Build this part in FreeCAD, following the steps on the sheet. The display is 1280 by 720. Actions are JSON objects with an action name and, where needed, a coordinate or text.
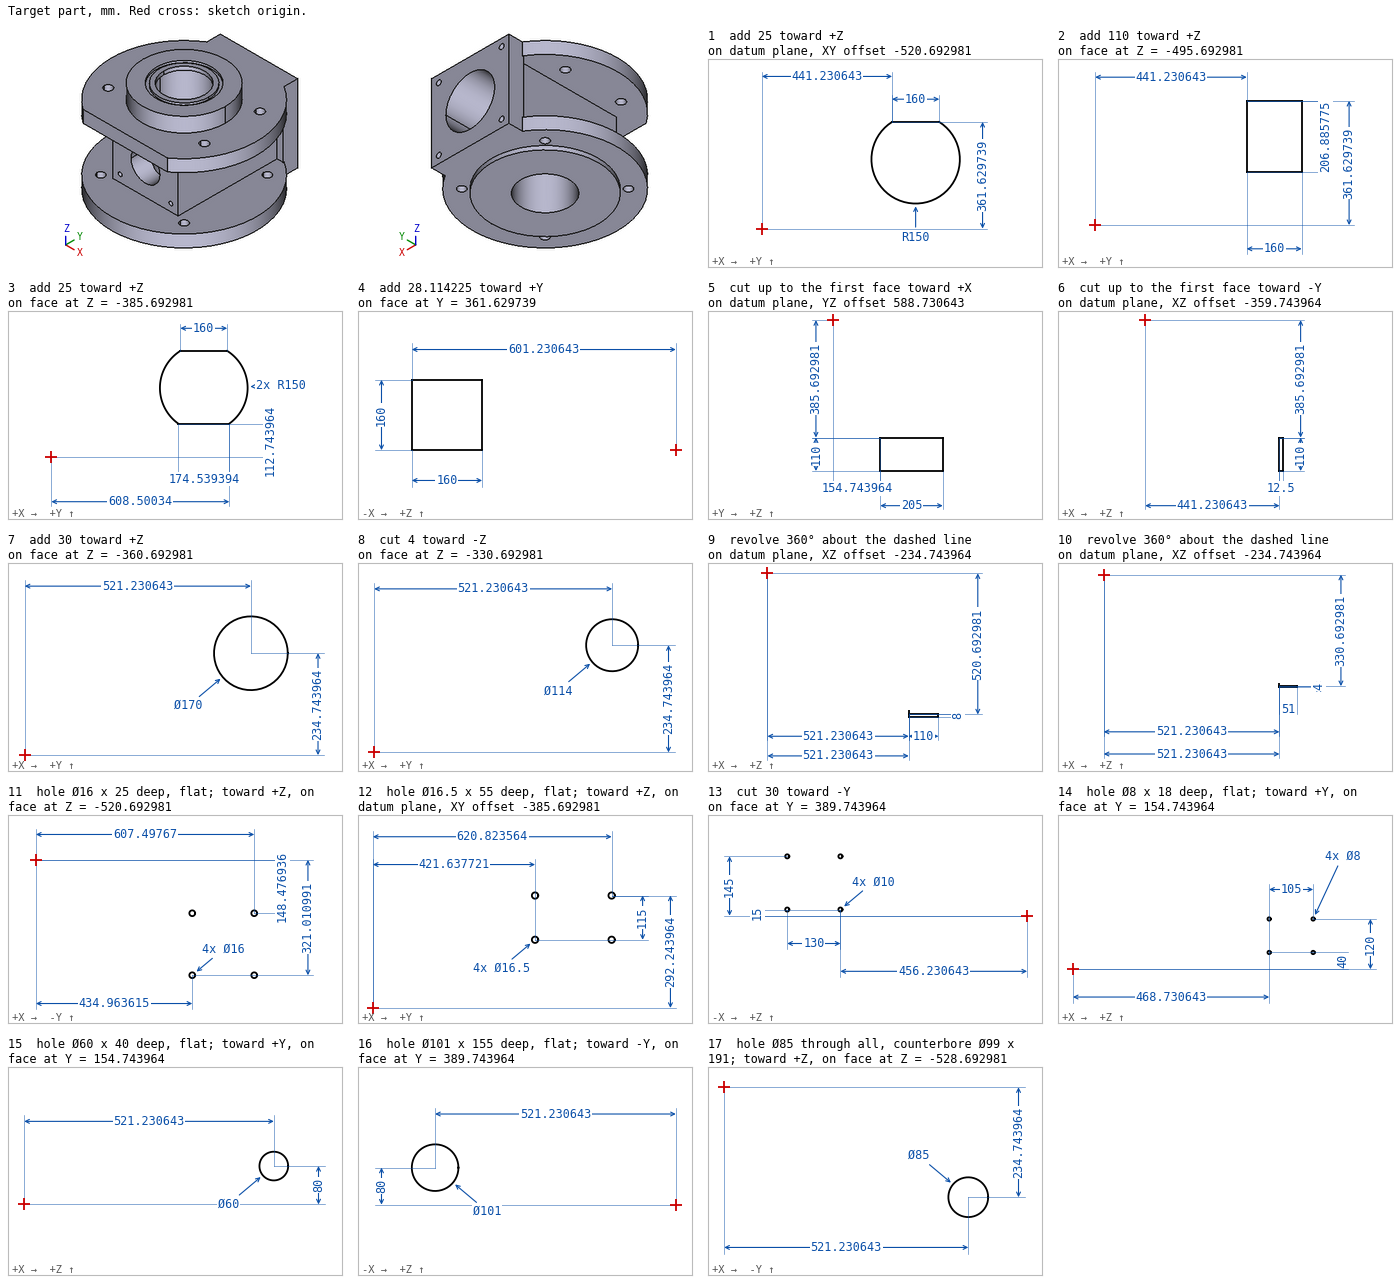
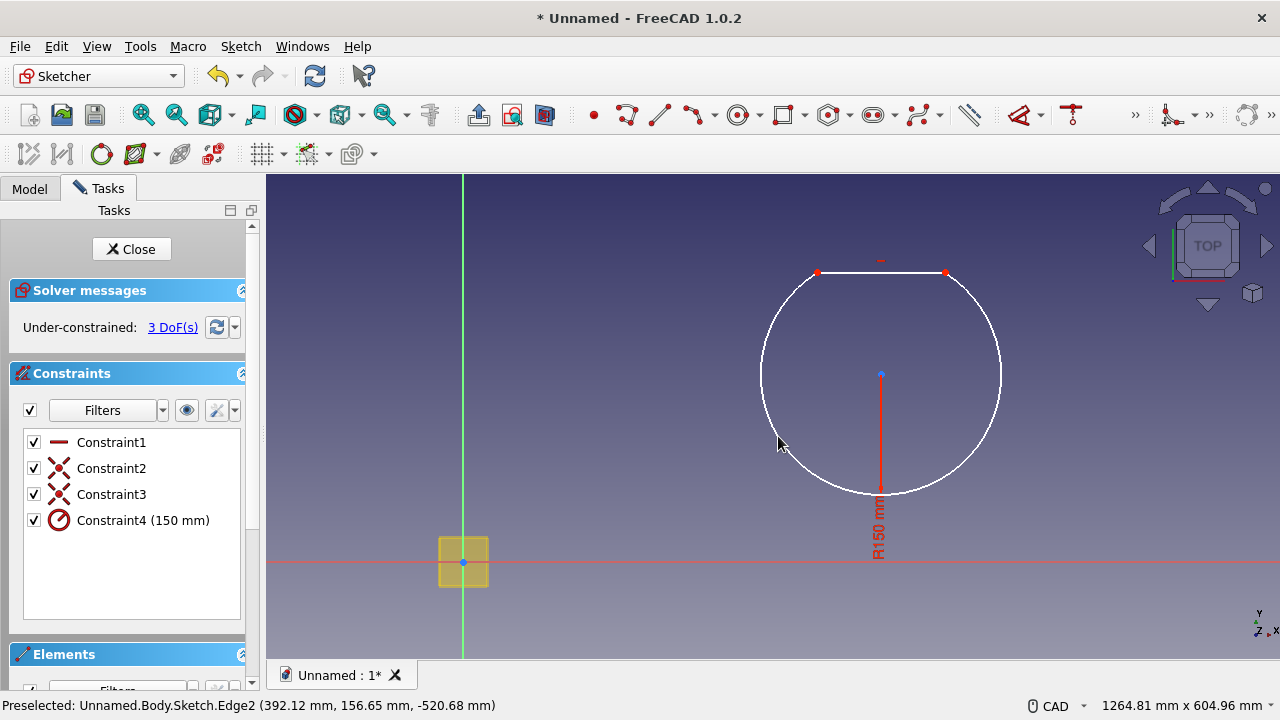
{"action": "left_click", "coordinate": [855, 273]}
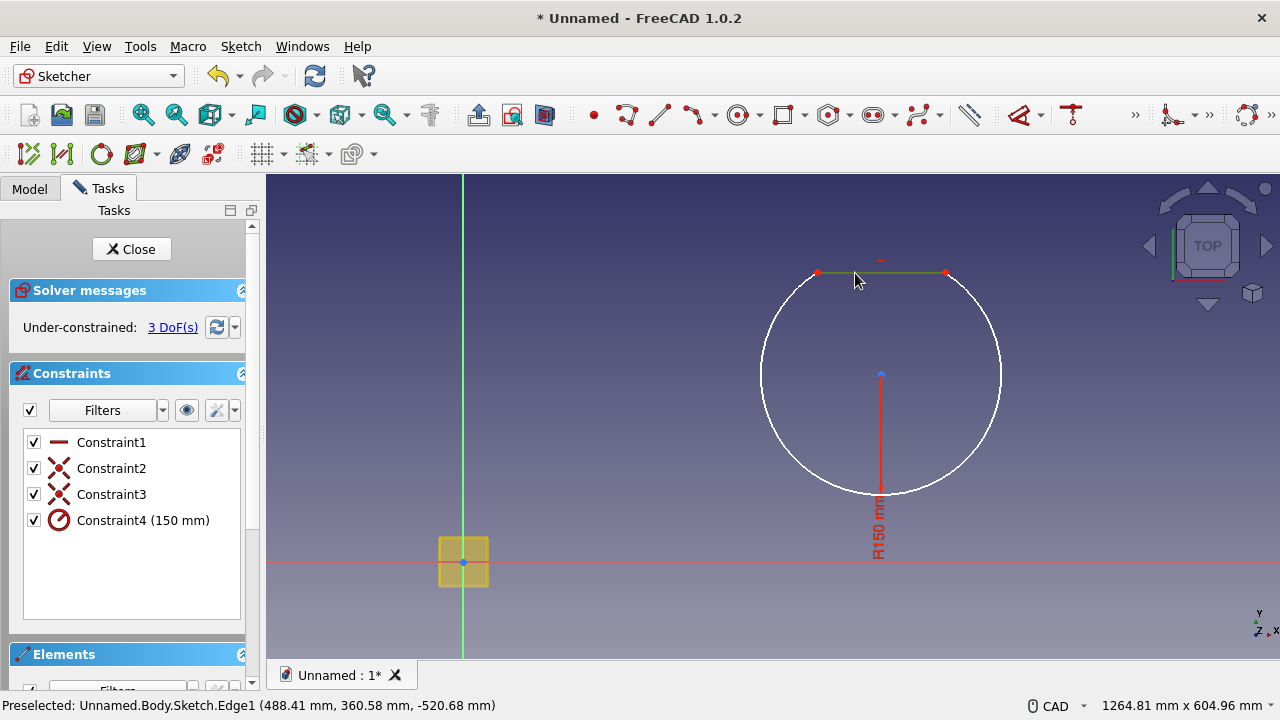
{"action": "left_click", "coordinate": [1040, 116]}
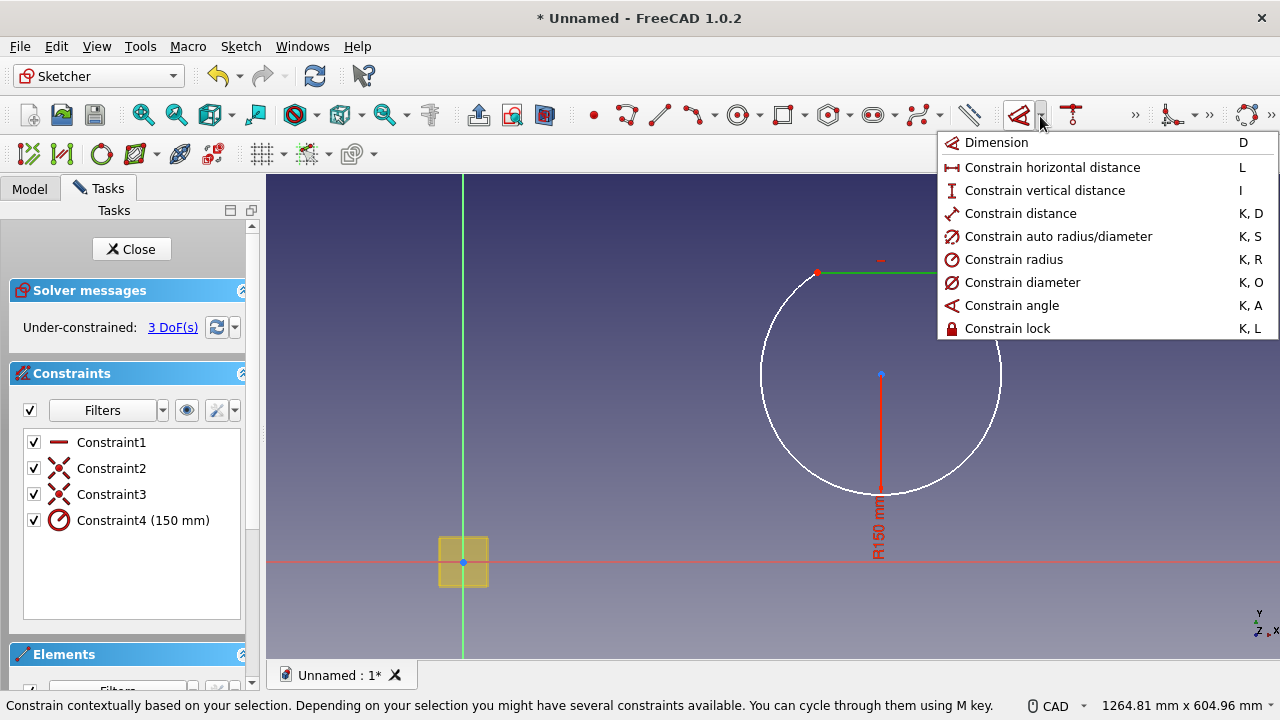
{"action": "left_click", "coordinate": [1108, 168]}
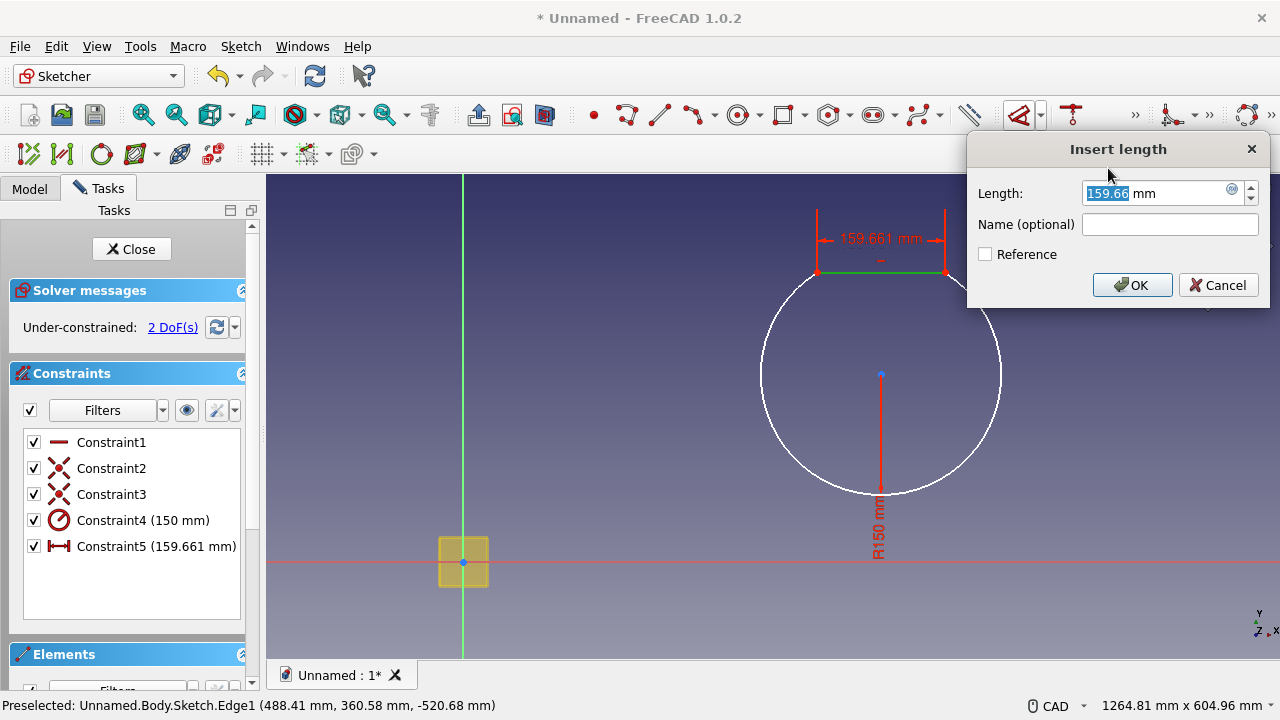
{"action": "type", "text": "160"}
{"action": "key", "text": "Return"}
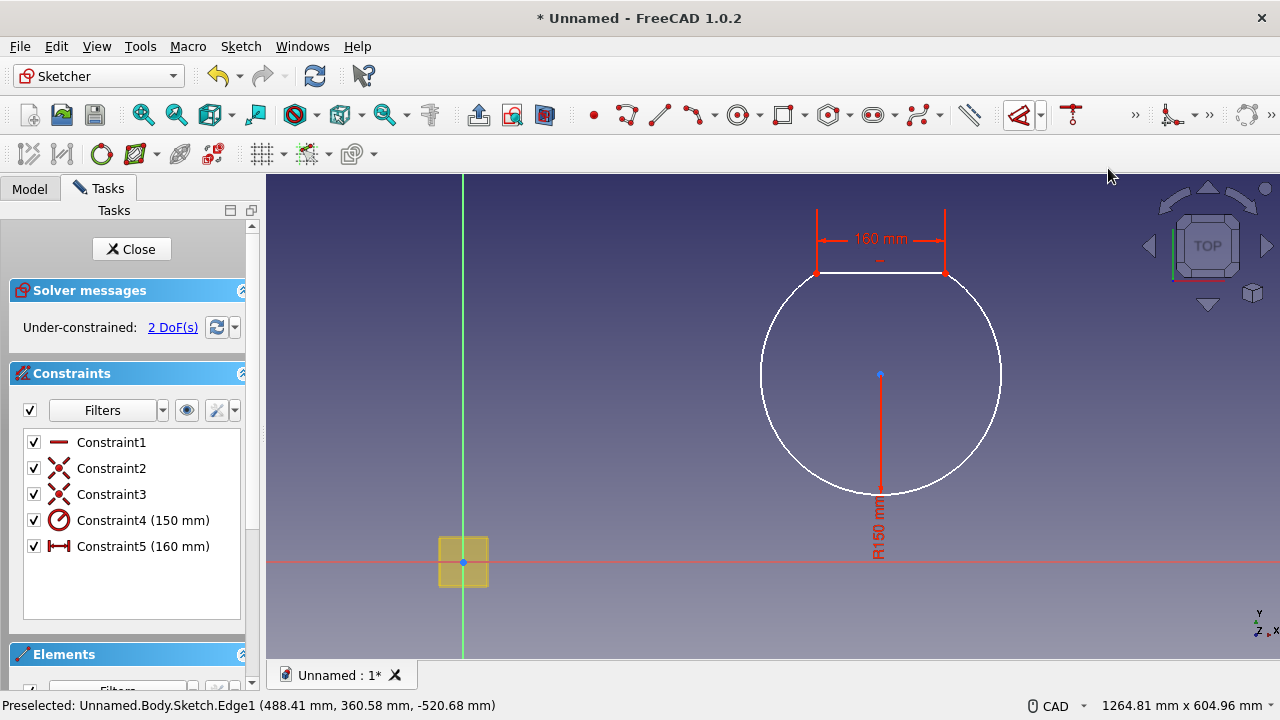
{"action": "left_click", "coordinate": [817, 273]}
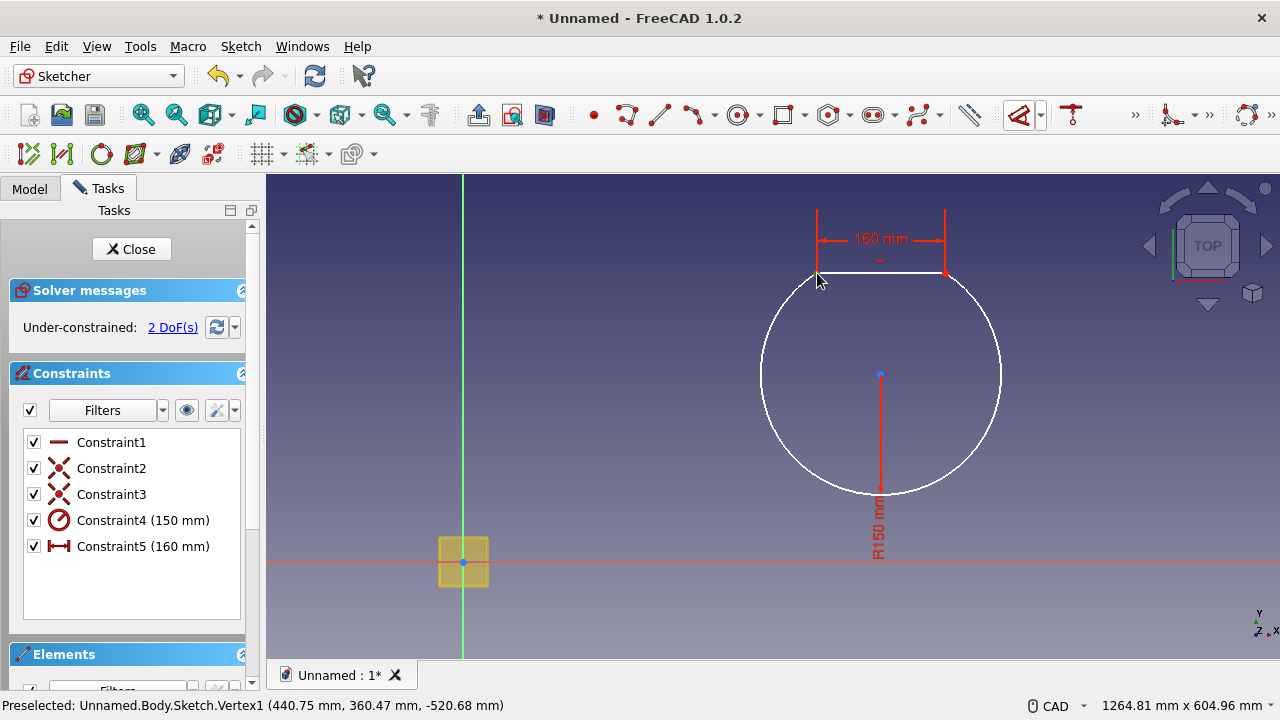
{"action": "left_click", "coordinate": [1040, 116]}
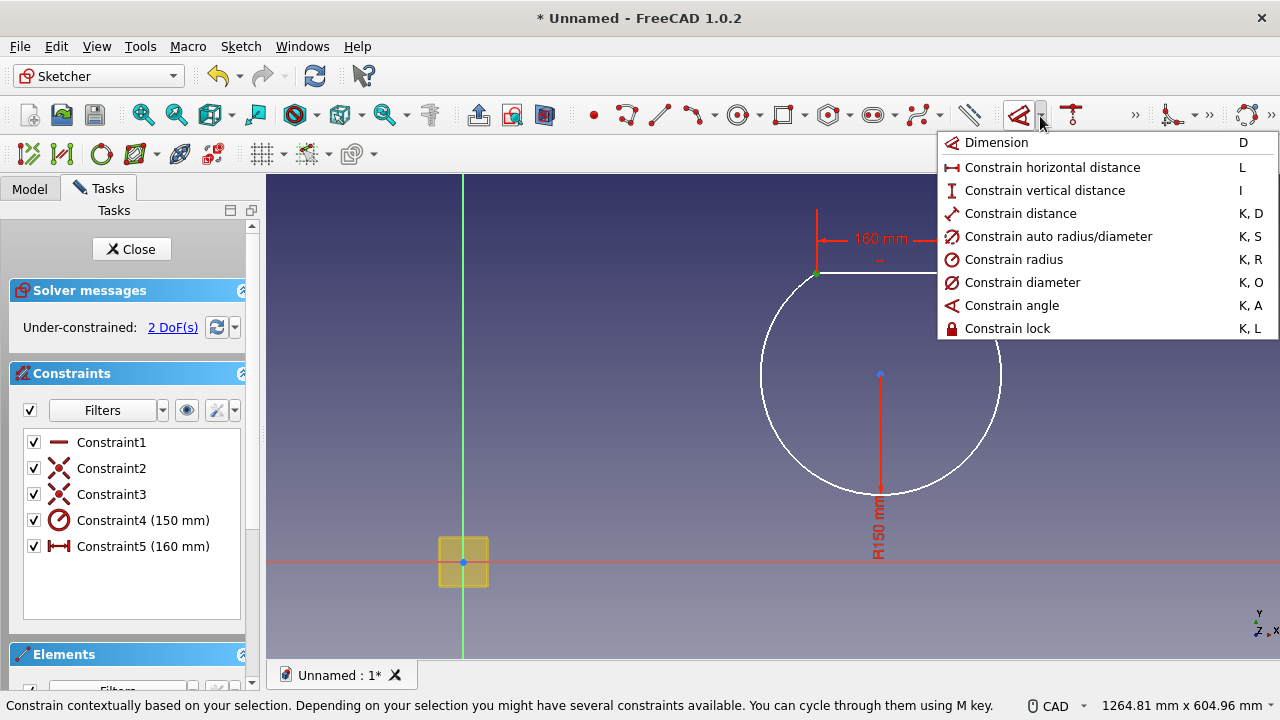
{"action": "left_click", "coordinate": [1108, 168]}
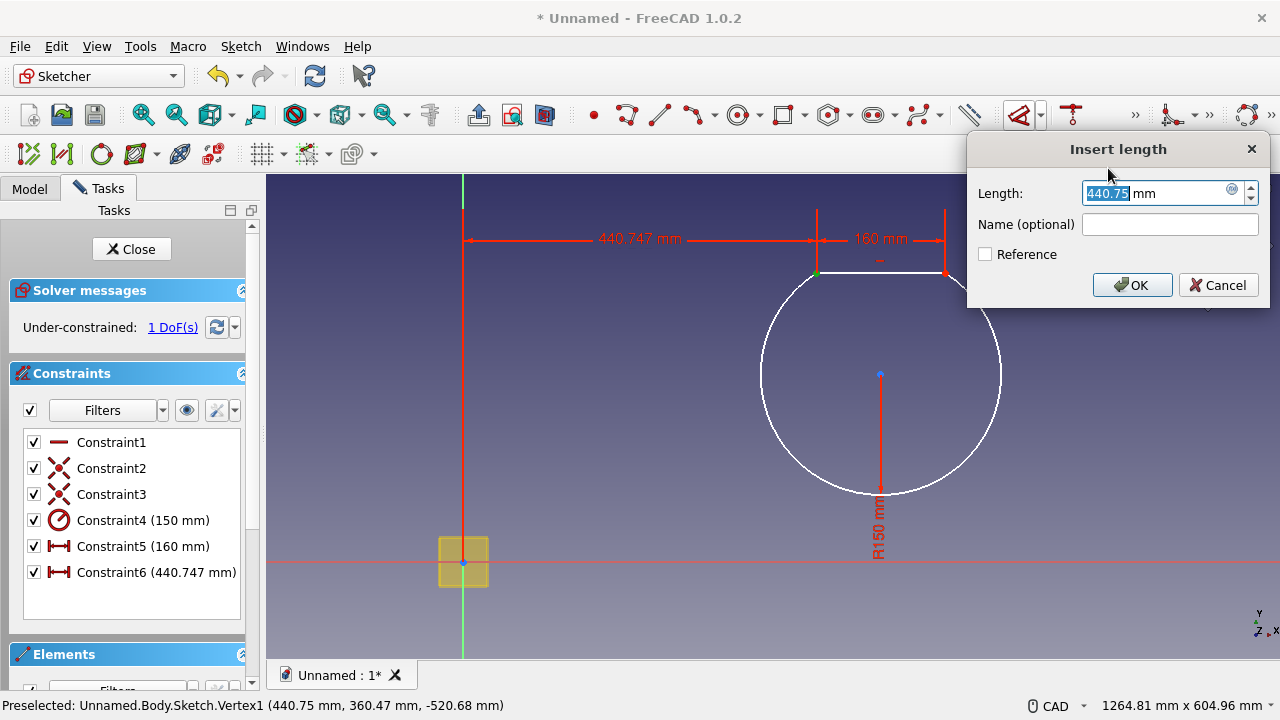
{"action": "type", "text": "441.230643"}
{"action": "key", "text": "Return"}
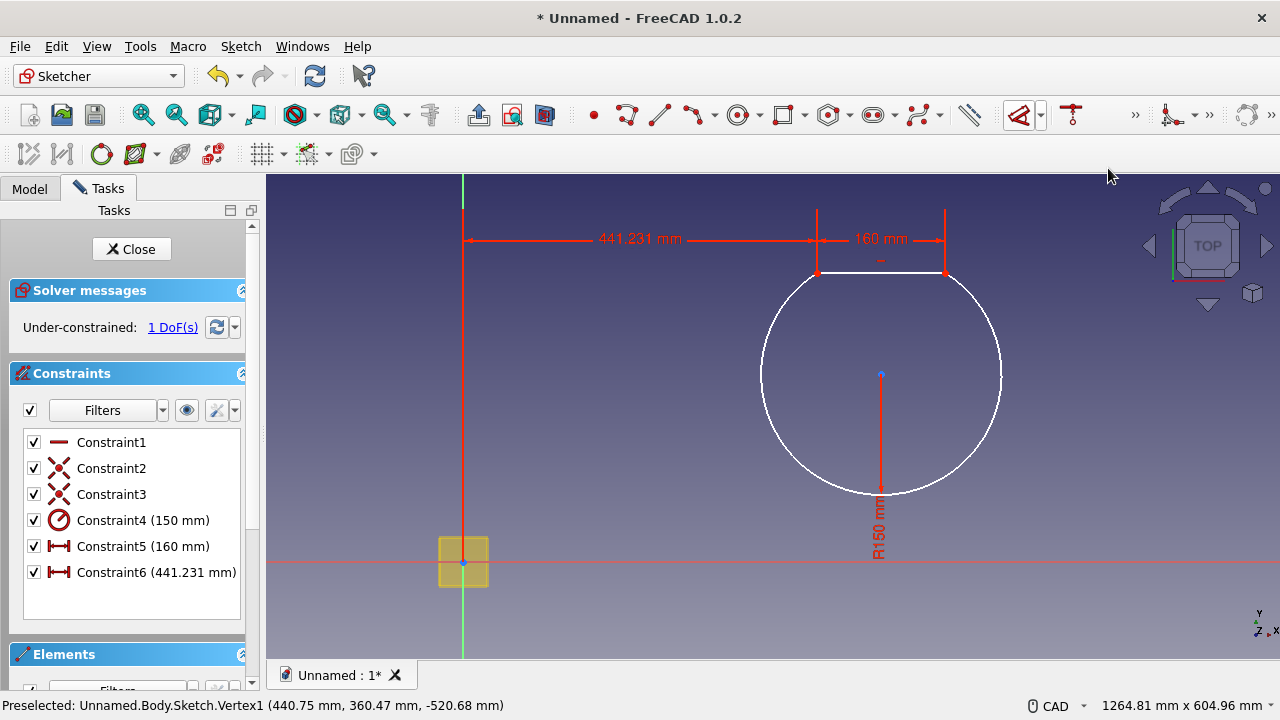
{"action": "left_click", "coordinate": [817, 273]}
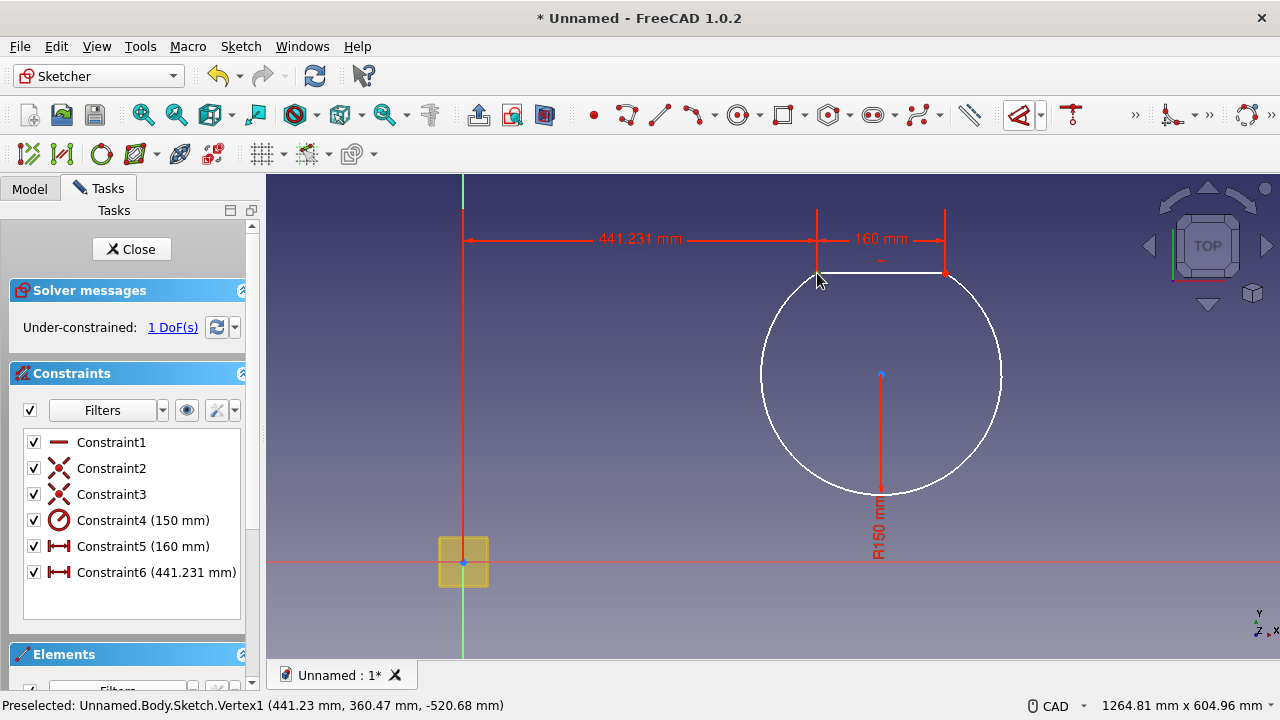
{"action": "left_click", "coordinate": [1040, 116]}